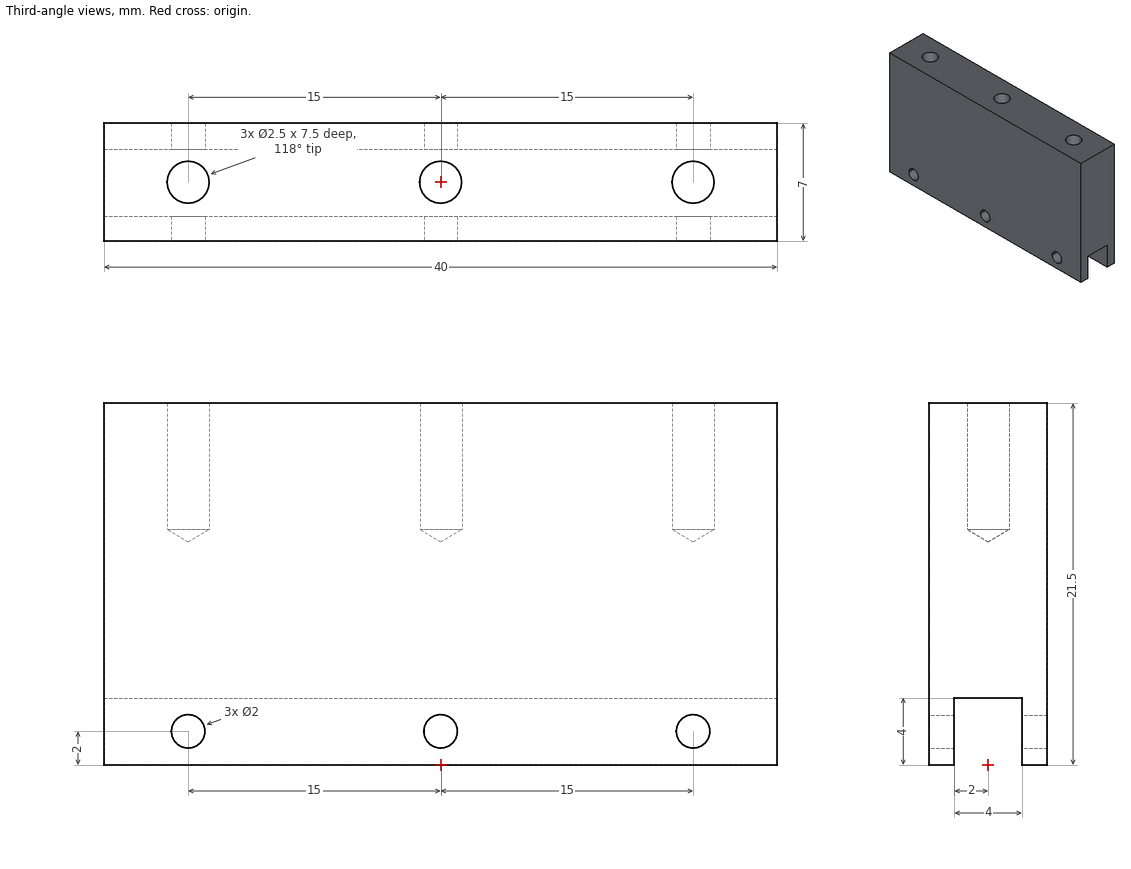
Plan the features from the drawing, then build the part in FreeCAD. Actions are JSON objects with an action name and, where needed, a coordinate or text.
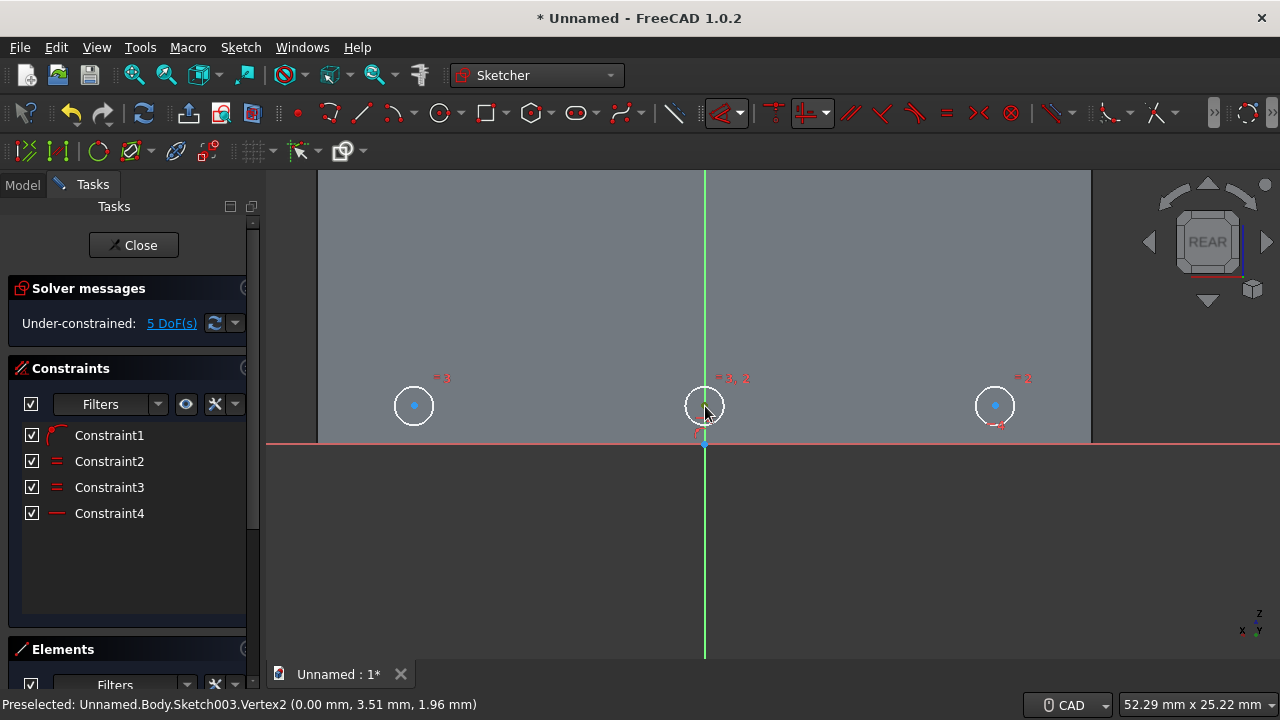
{"action": "left_click", "coordinate": [414, 406]}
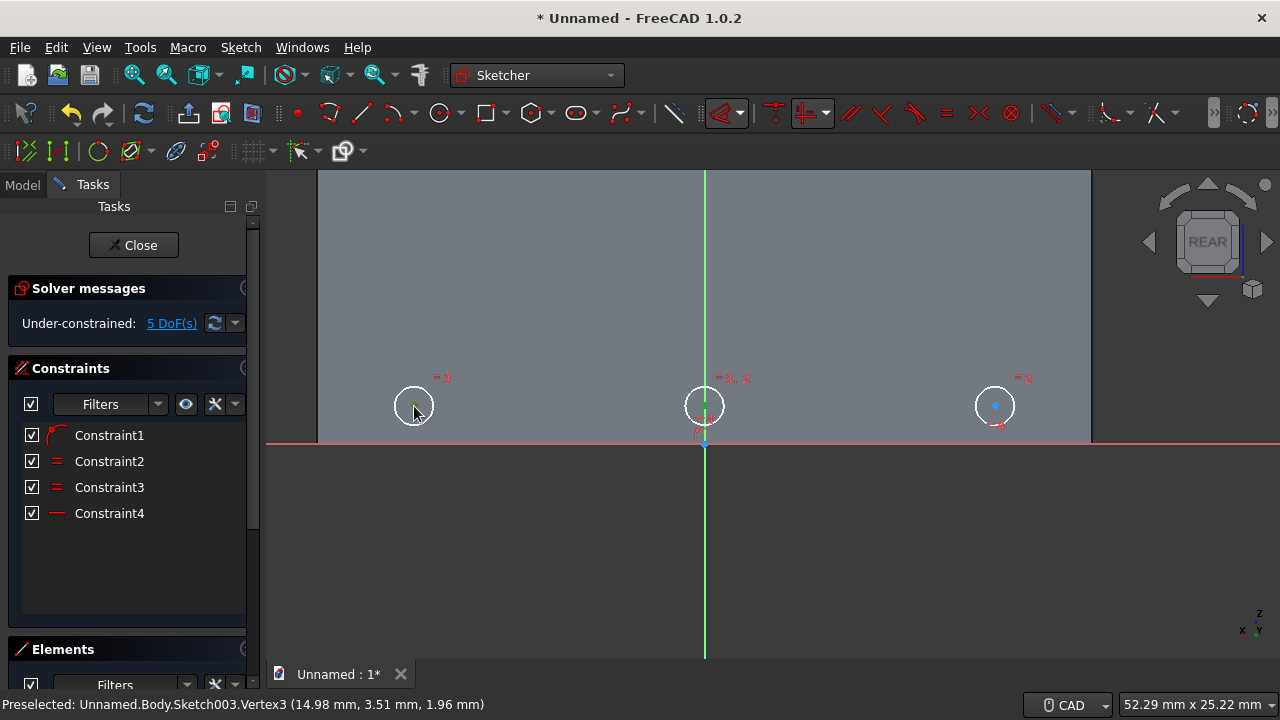
{"action": "left_click", "coordinate": [828, 114]}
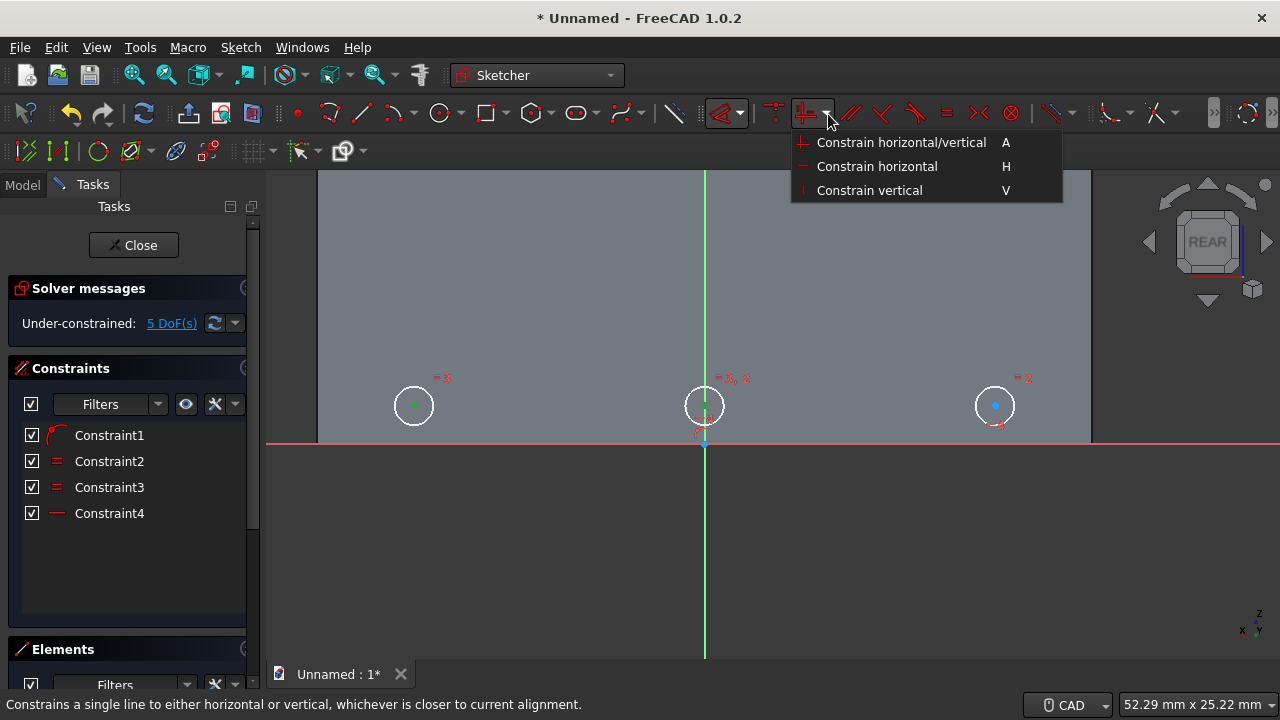
{"action": "left_click", "coordinate": [927, 166]}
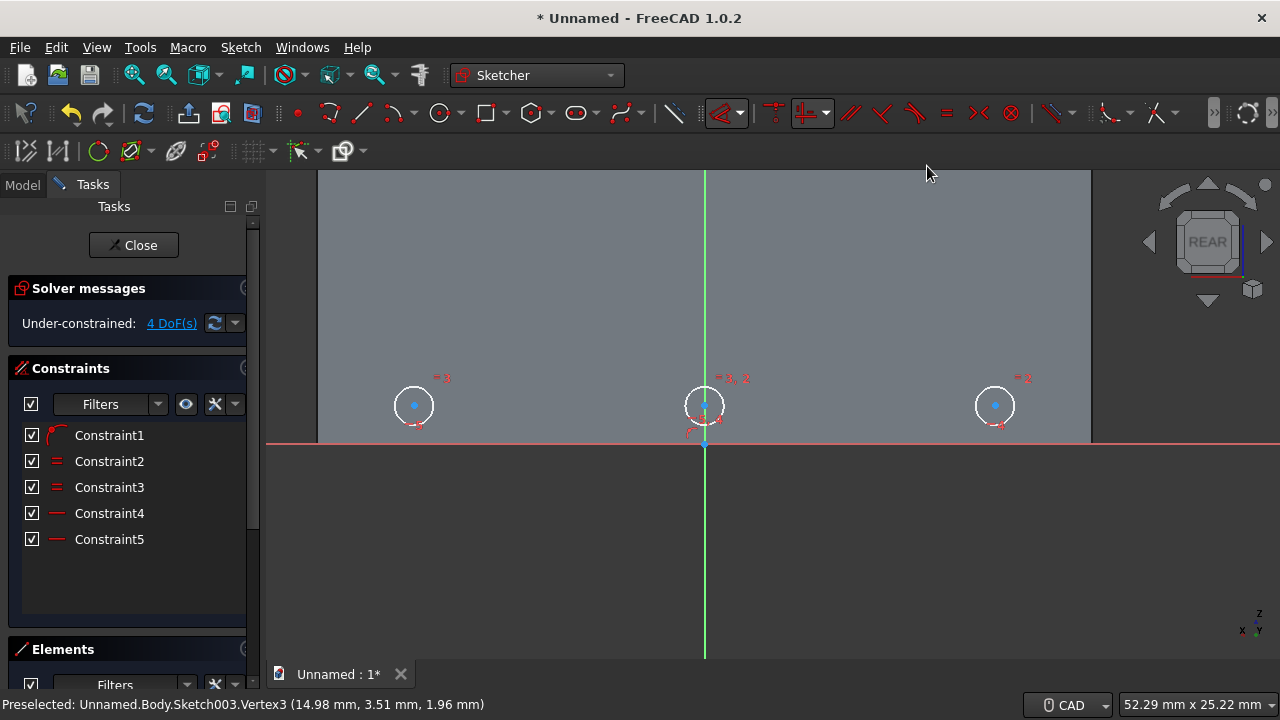
{"action": "left_click", "coordinate": [1008, 392]}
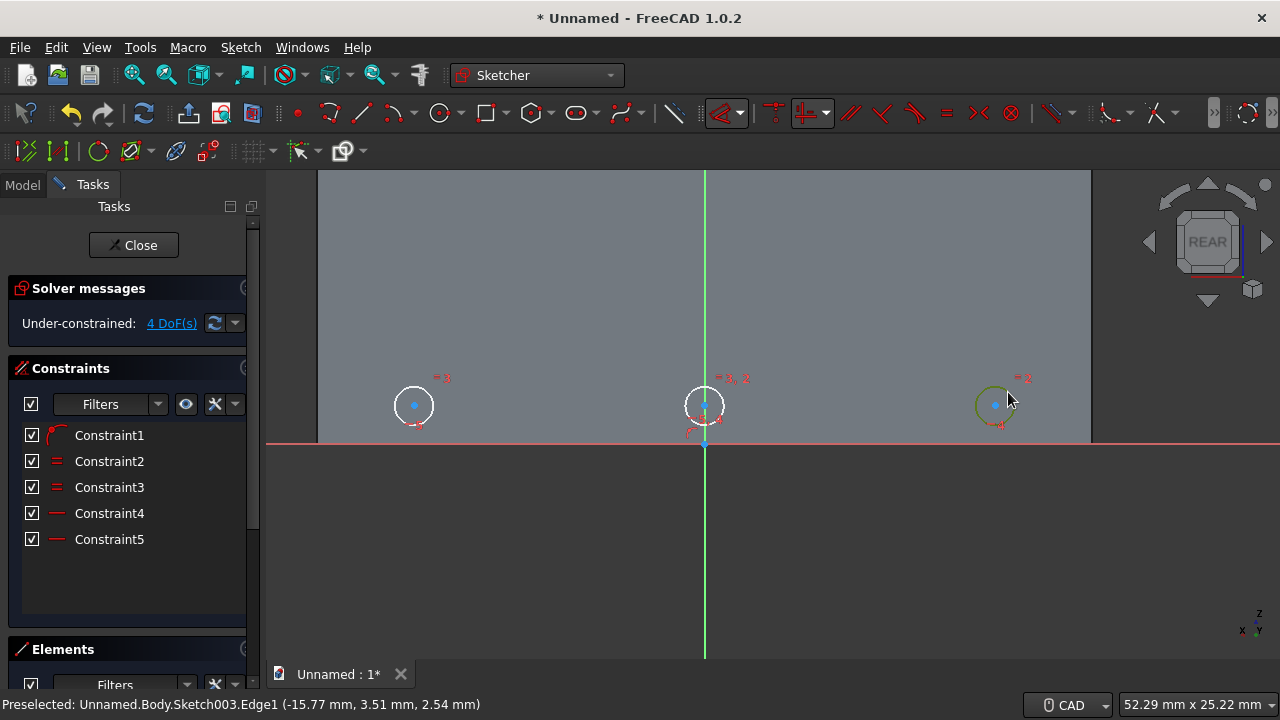
{"action": "key", "text": "k o"}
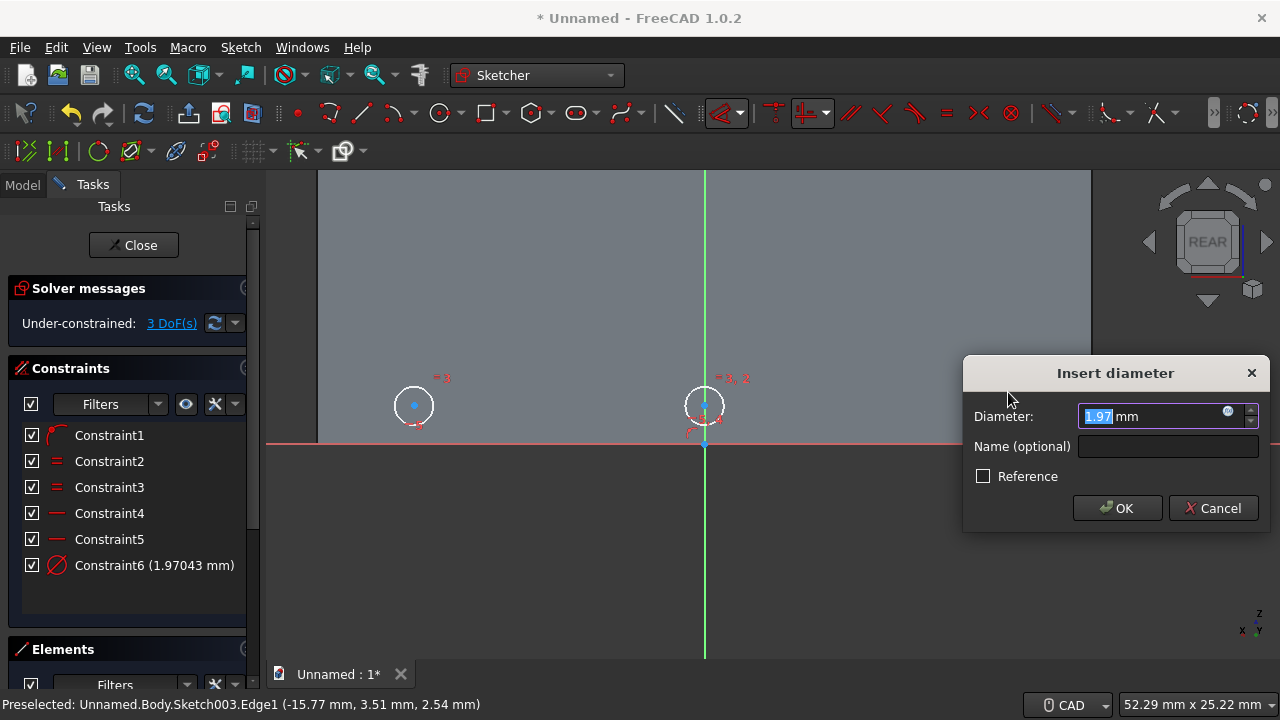
{"action": "type", "text": "2"}
{"action": "key", "text": "Return"}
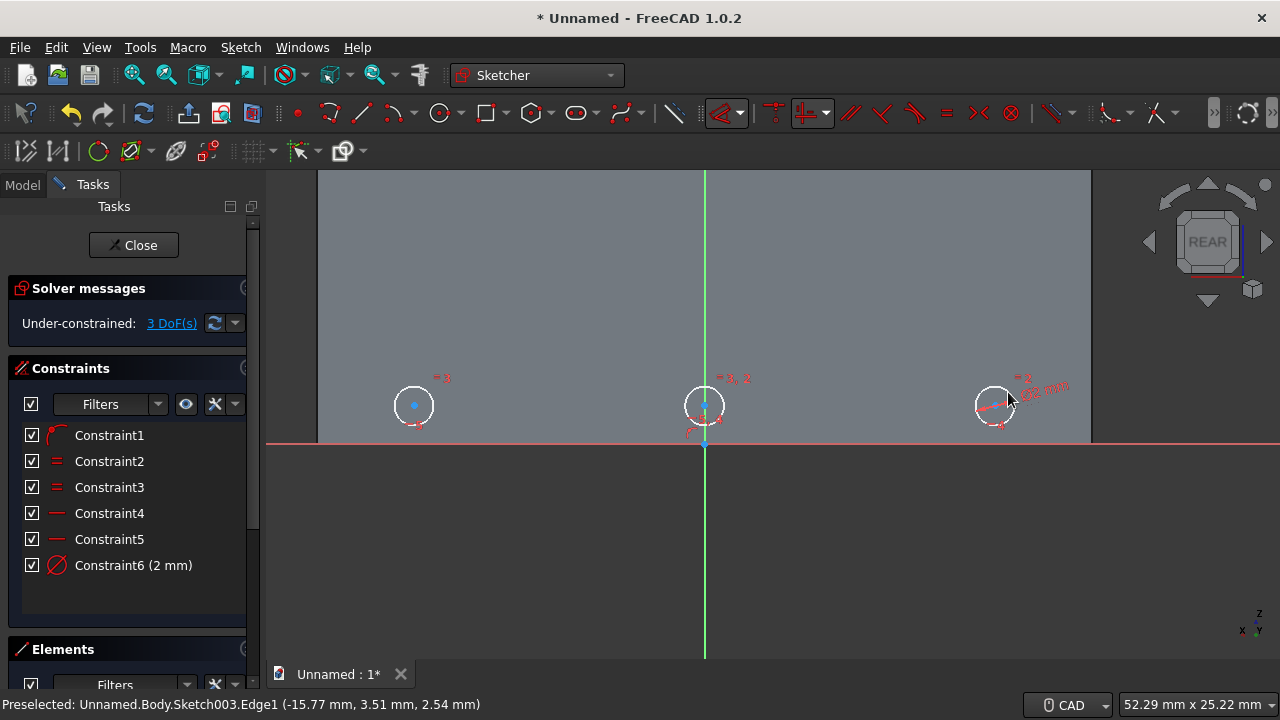
{"action": "left_click", "coordinate": [995, 406]}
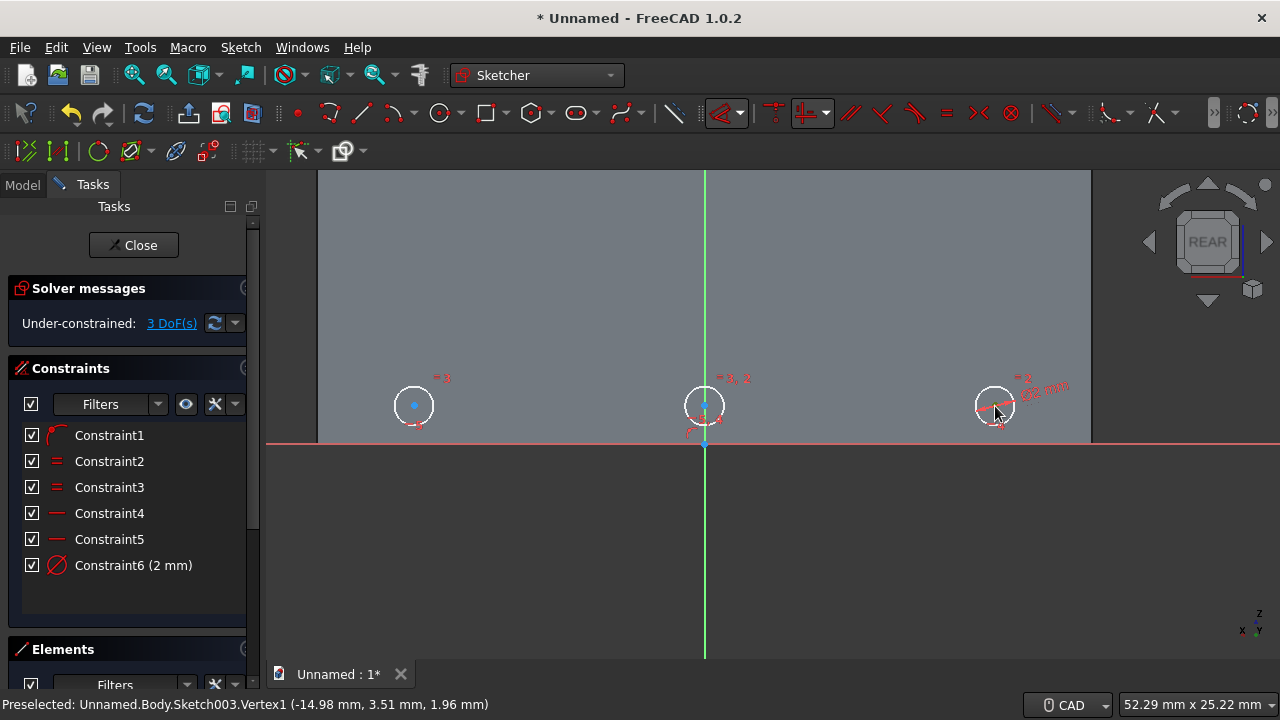
{"action": "key", "text": "i"}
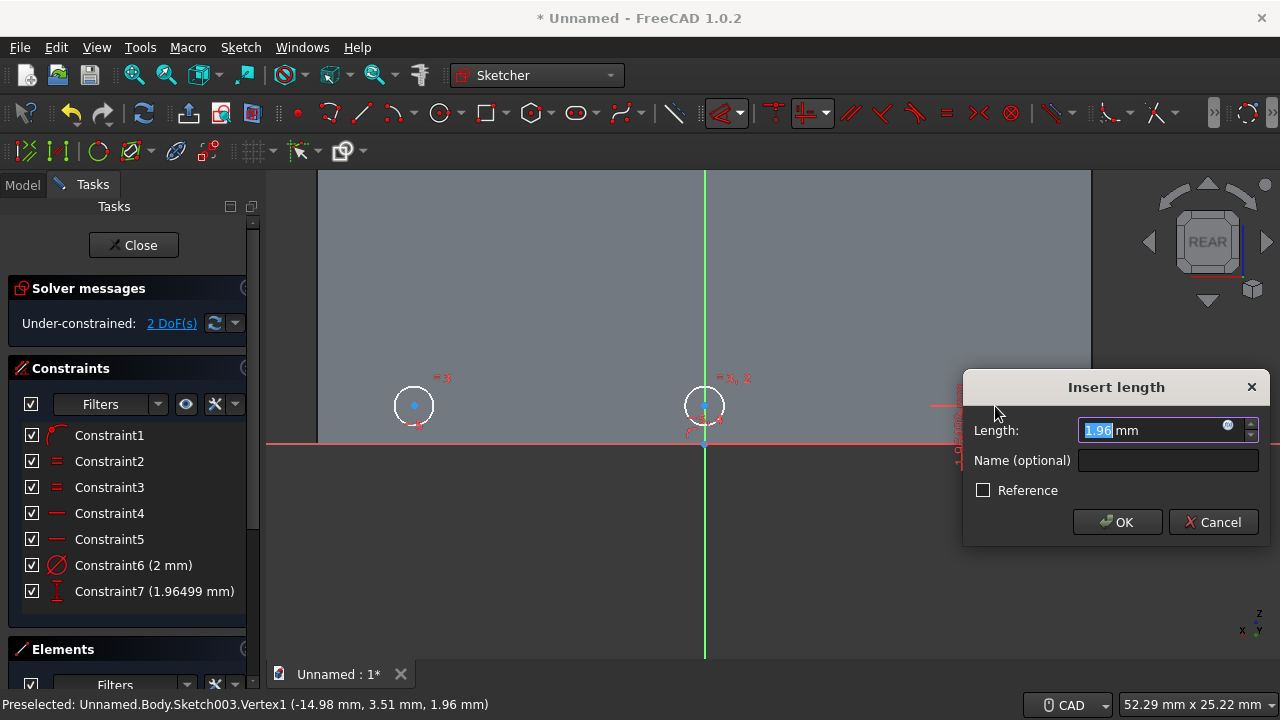
{"action": "type", "text": "2"}
{"action": "key", "text": "Return"}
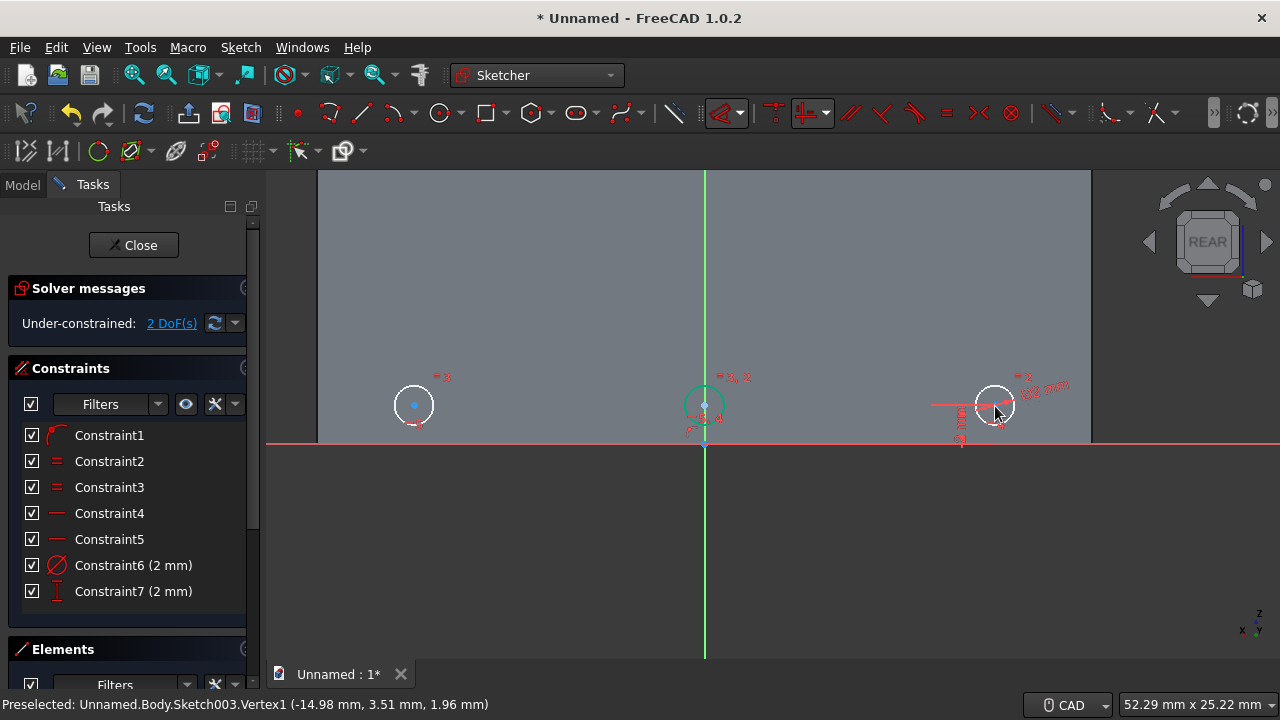
{"action": "left_click", "coordinate": [995, 405]}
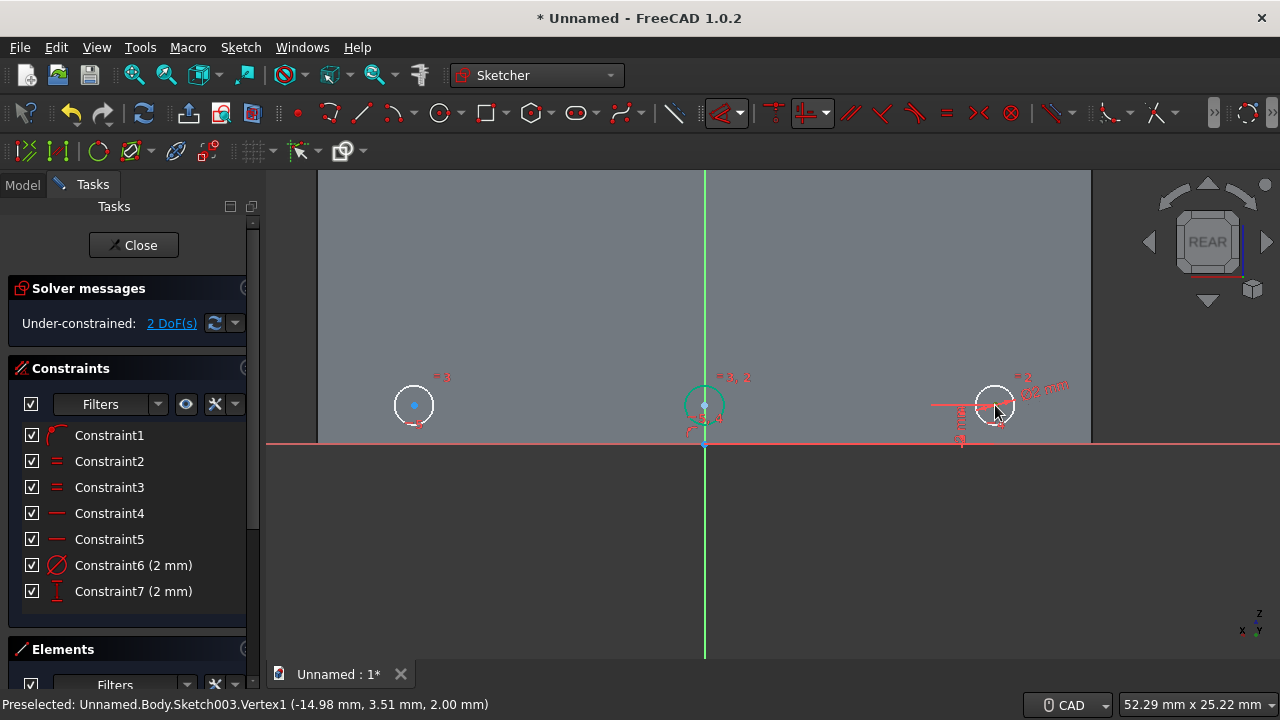
{"action": "key", "text": "l"}